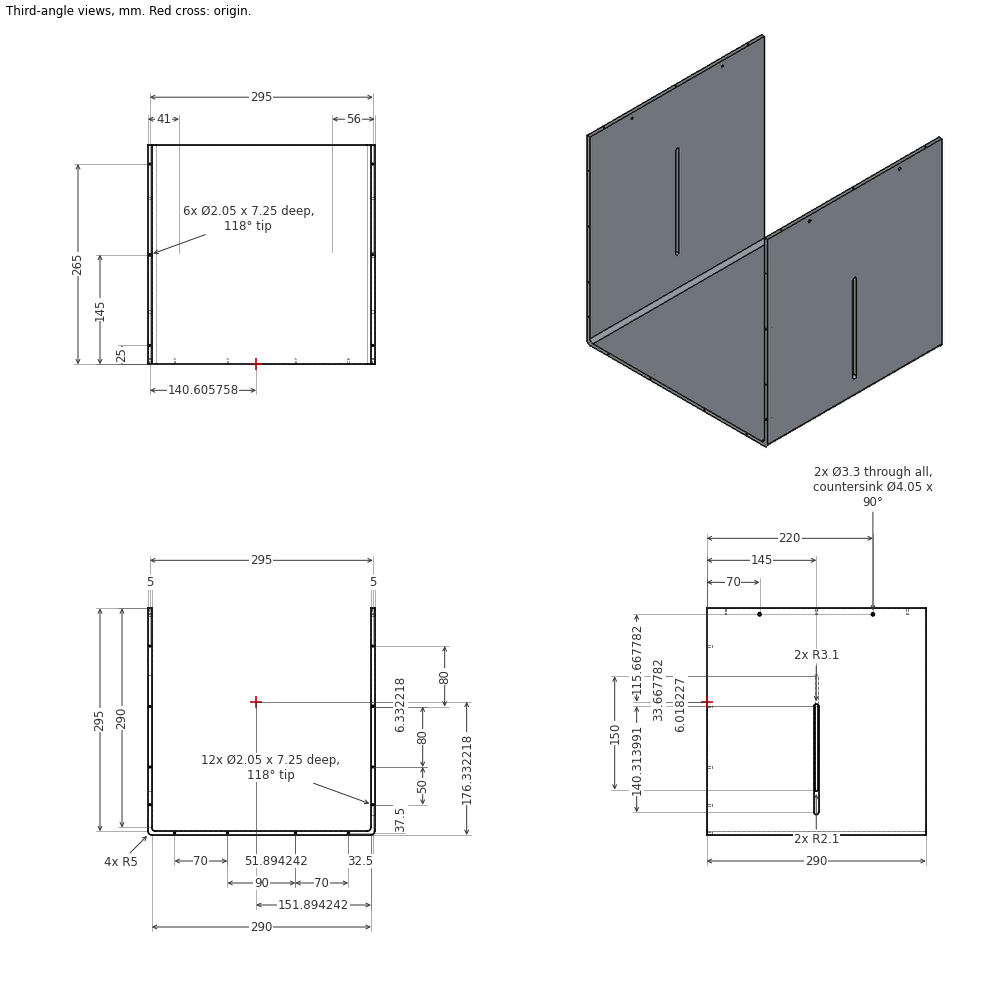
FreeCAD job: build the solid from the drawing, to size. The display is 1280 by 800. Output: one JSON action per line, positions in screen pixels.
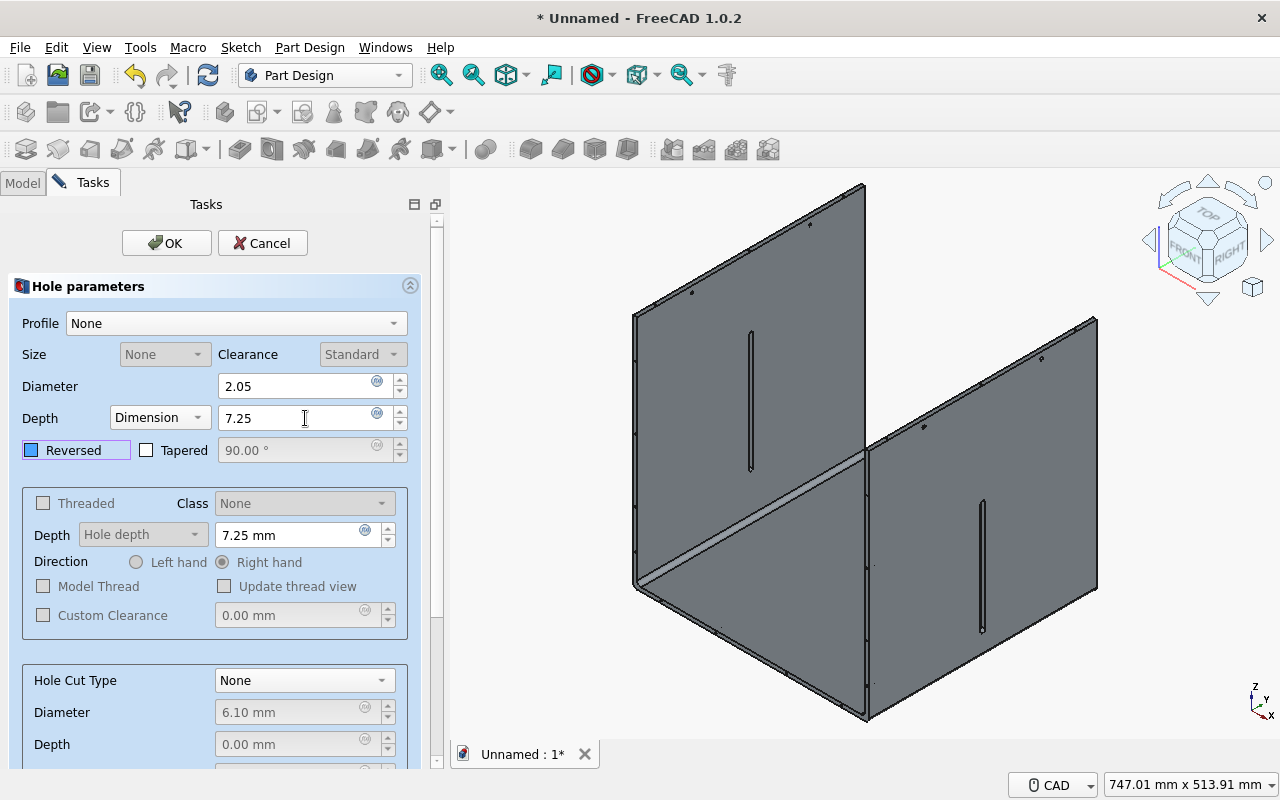
{"action": "left_click", "coordinate": [167, 243]}